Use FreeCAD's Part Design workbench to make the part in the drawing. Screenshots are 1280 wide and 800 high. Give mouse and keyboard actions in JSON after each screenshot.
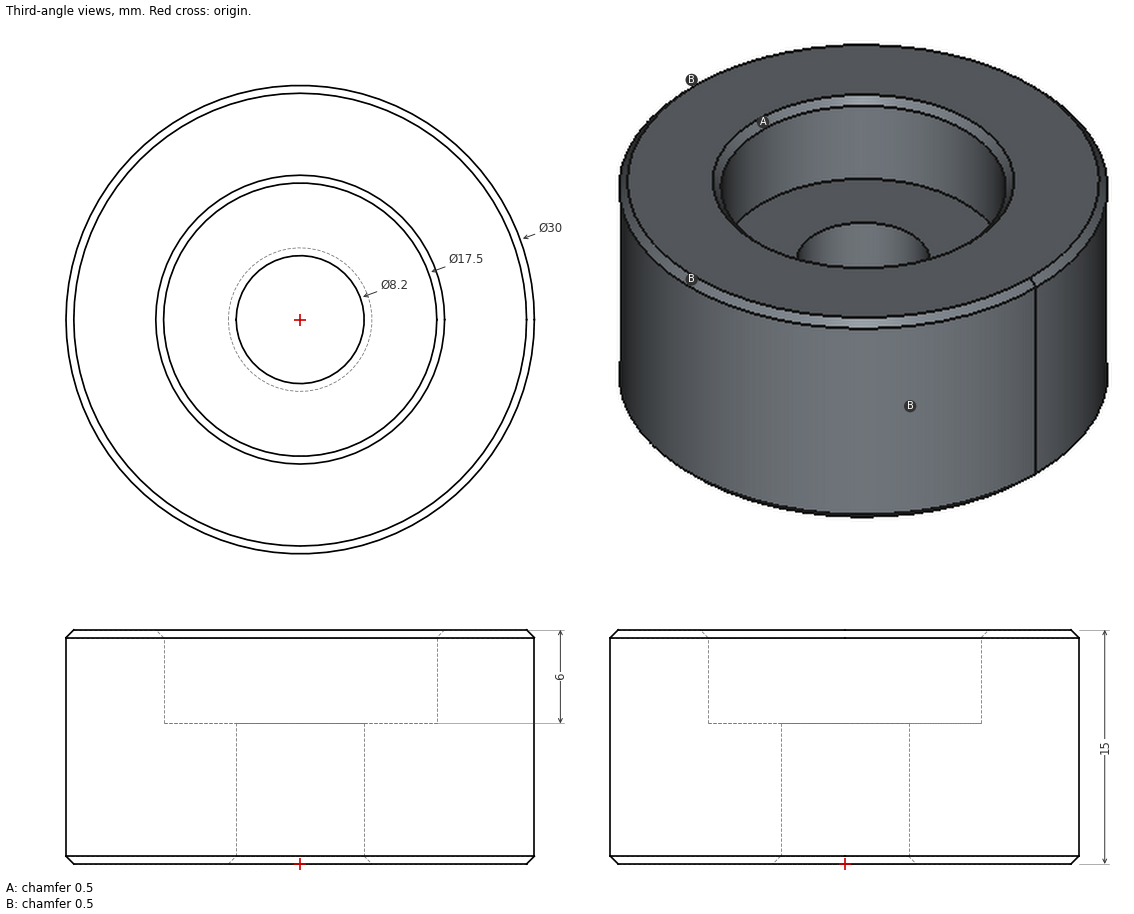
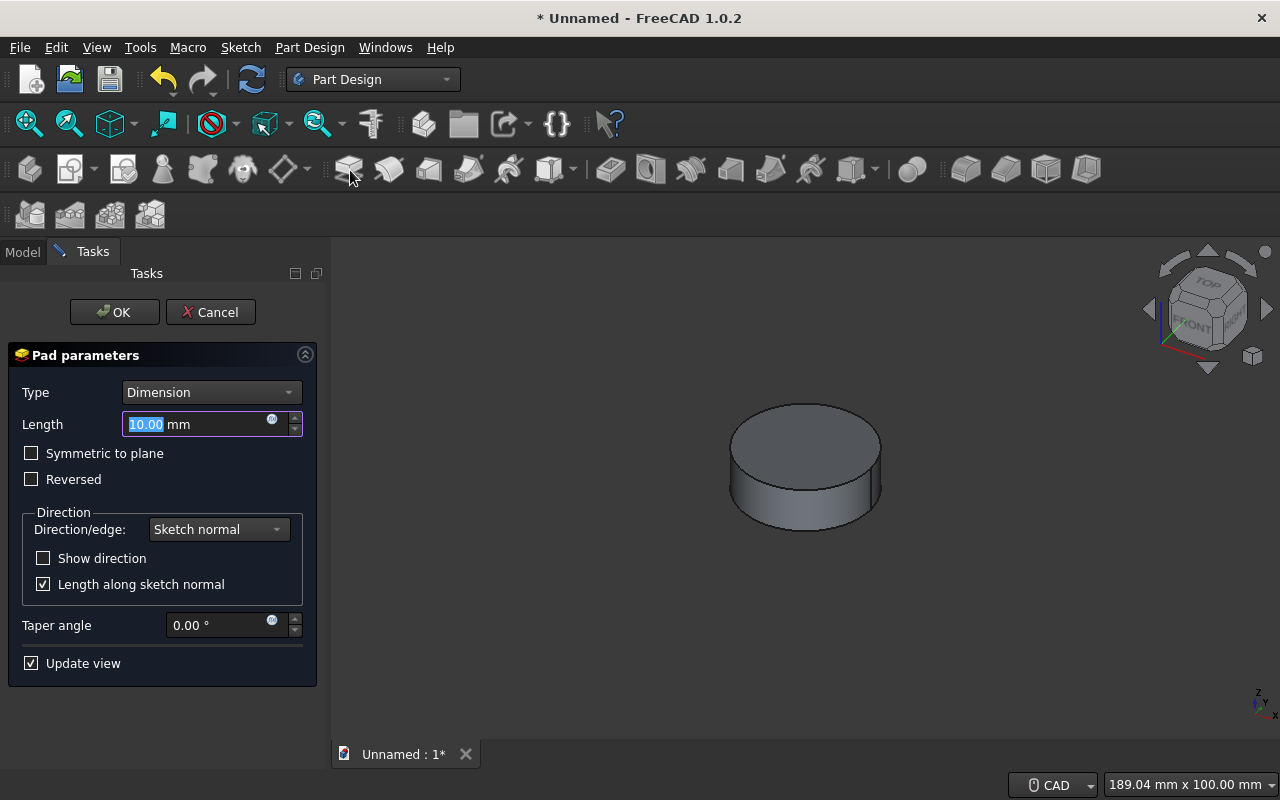
{"action": "type", "text": "15"}
{"action": "key", "text": "Tab"}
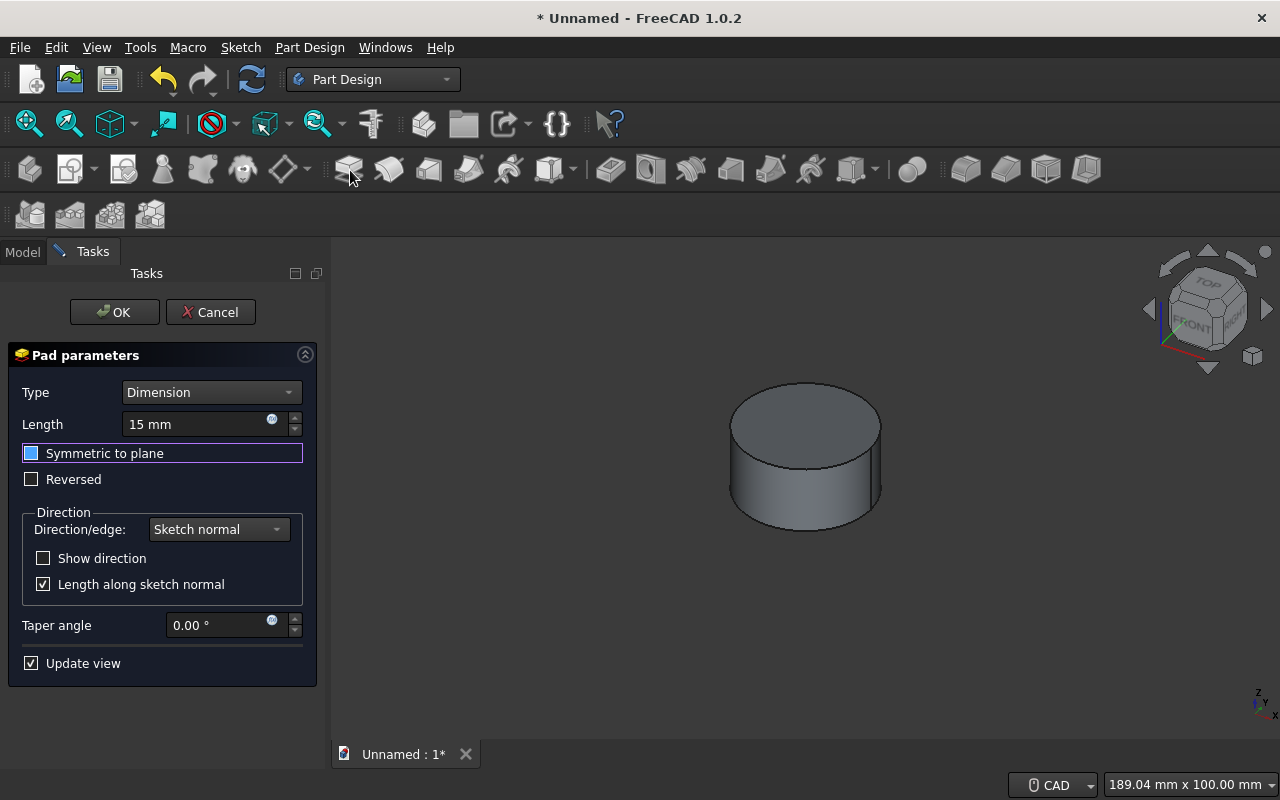
{"action": "left_click", "coordinate": [115, 312]}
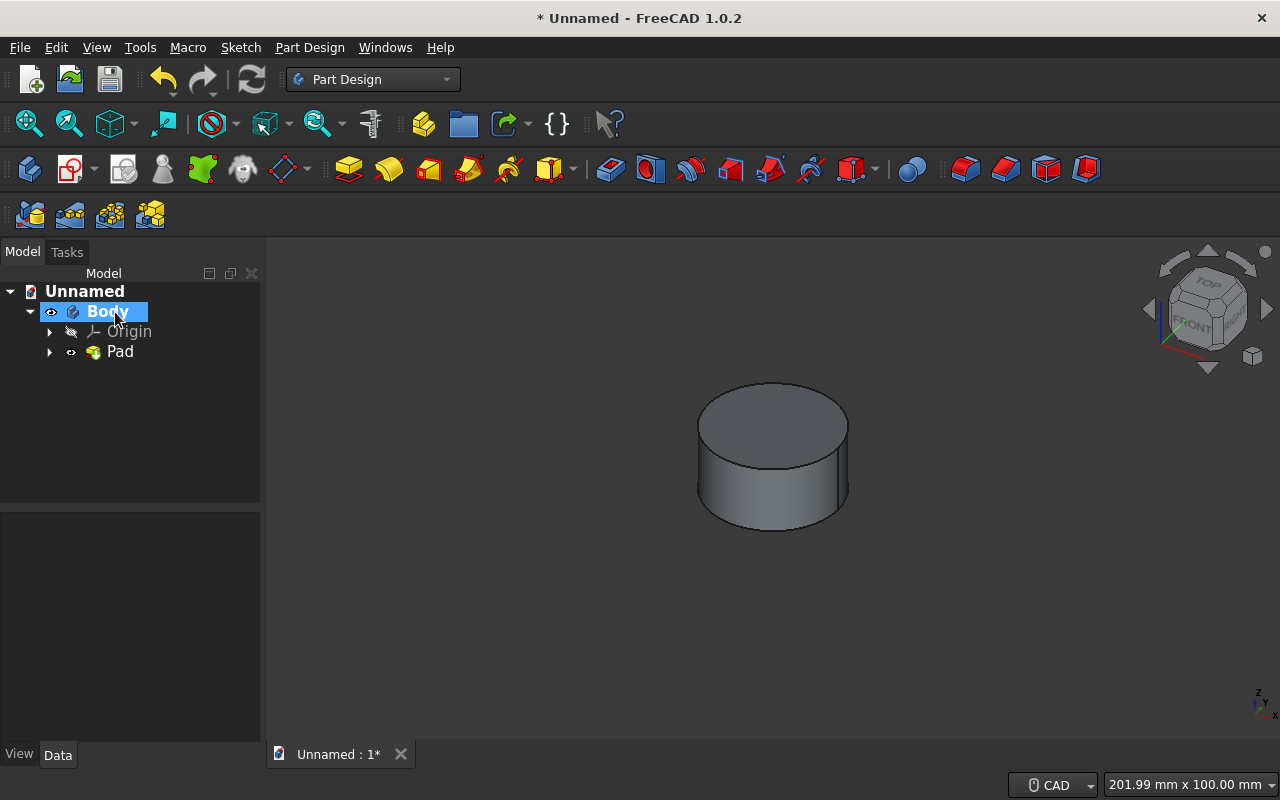
{"action": "left_click", "coordinate": [30, 124]}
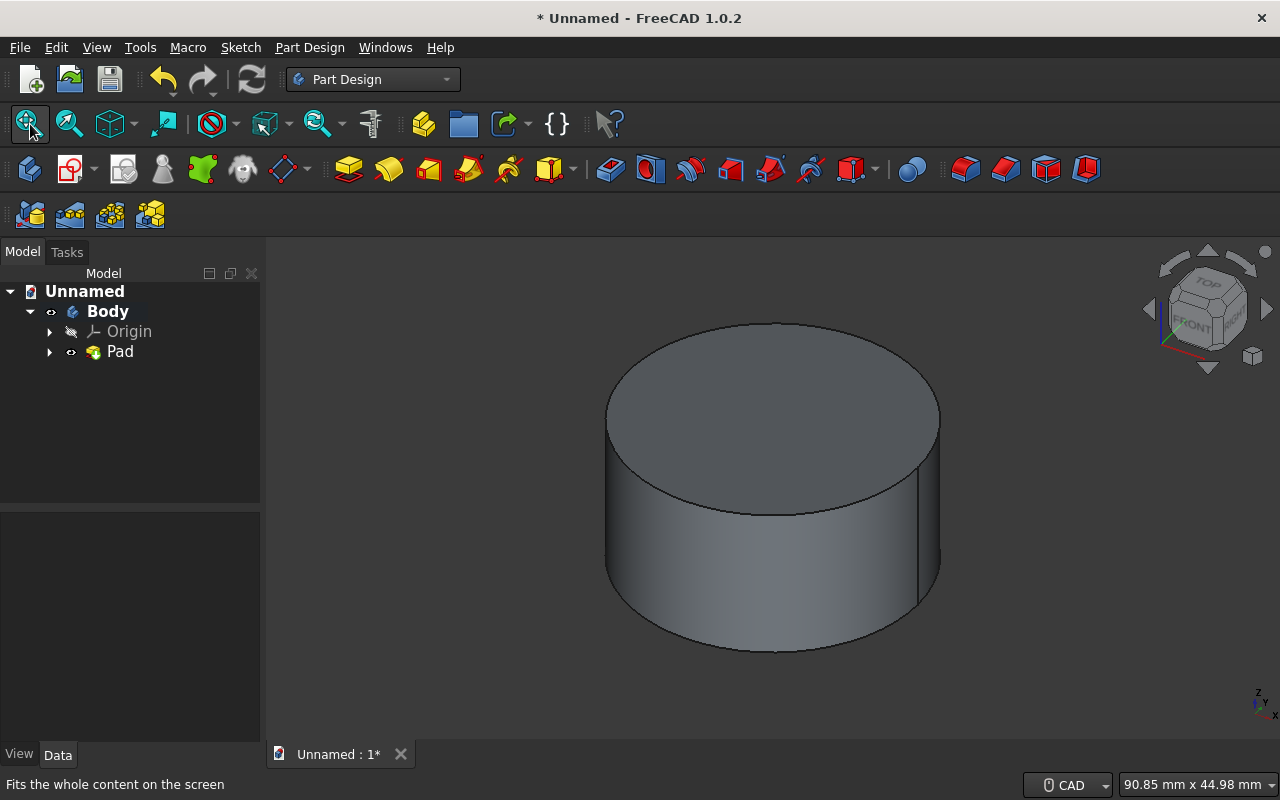
{"action": "left_click", "coordinate": [70, 170]}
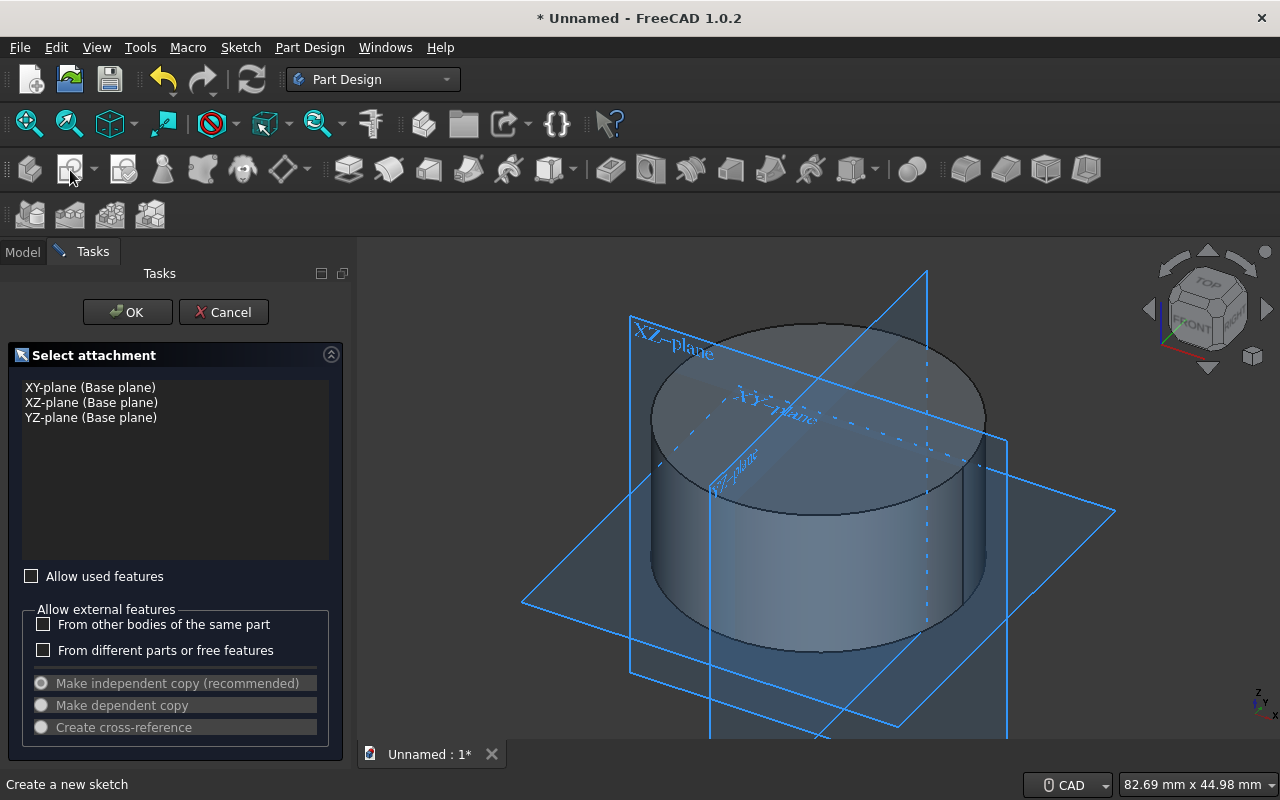
{"action": "left_click", "coordinate": [82, 388]}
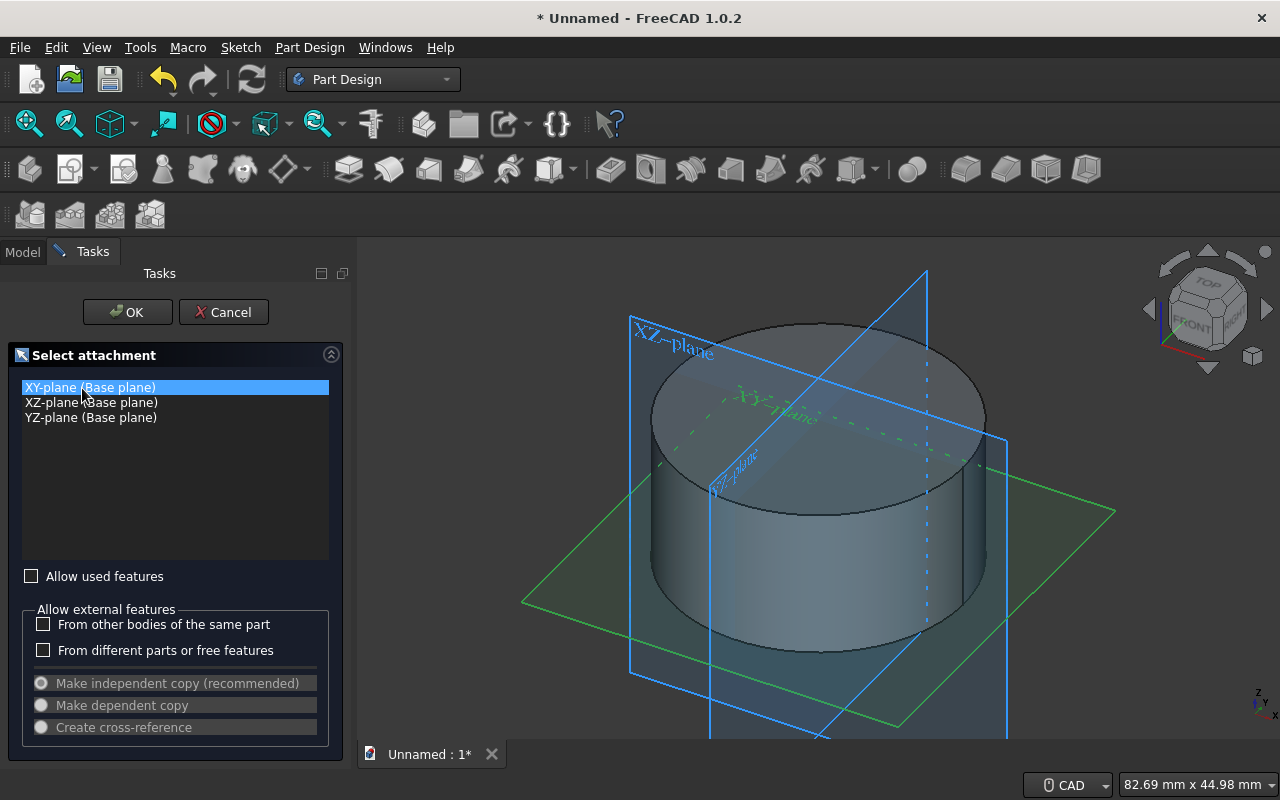
{"action": "left_click", "coordinate": [128, 312]}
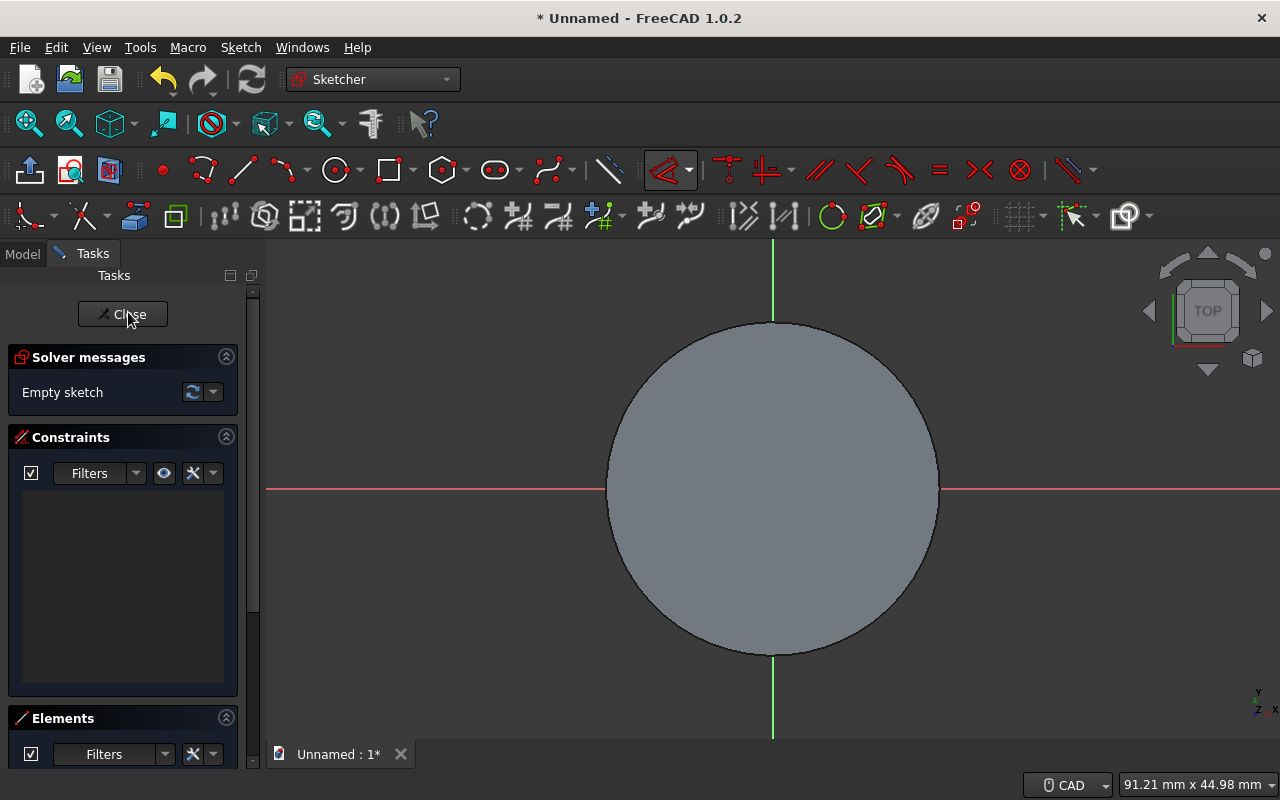
{"action": "key", "text": "q s"}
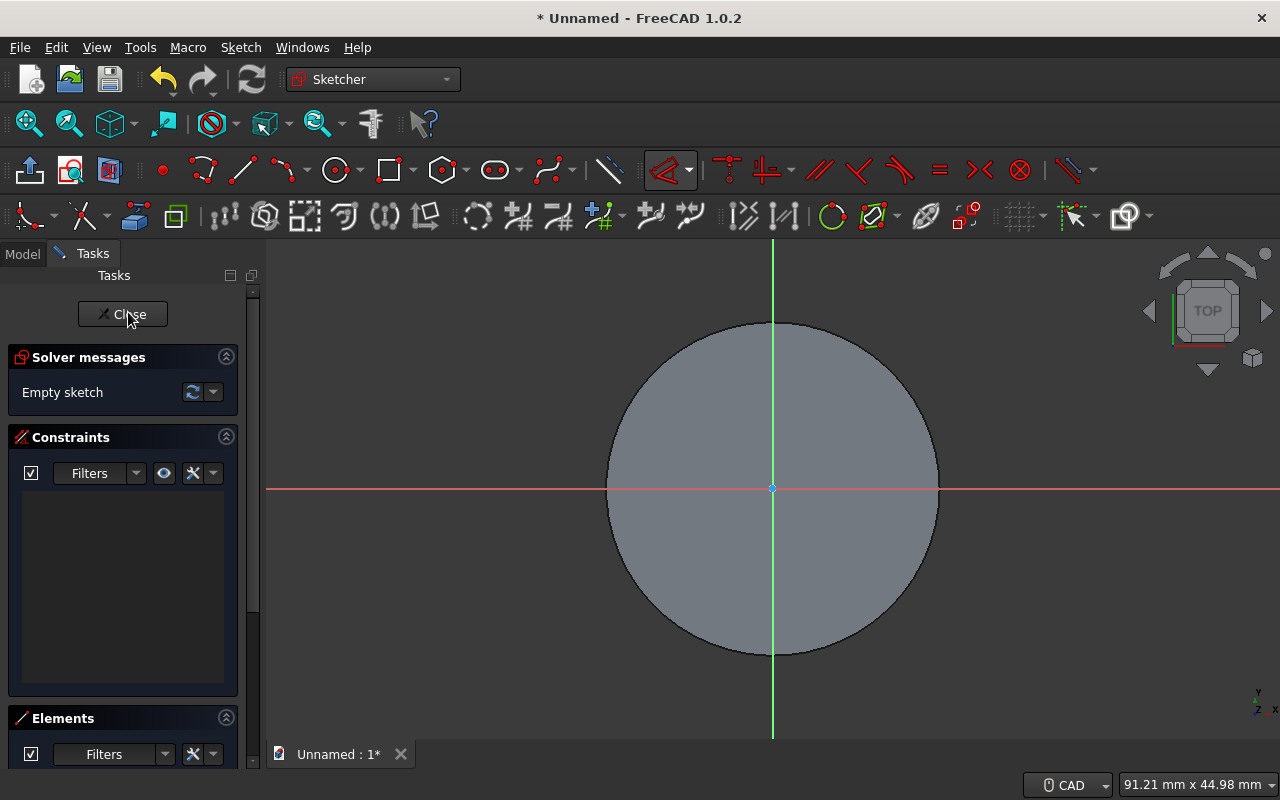
{"action": "scroll", "coordinate": [802, 489], "scroll_direction": "up", "scroll_amount": 6}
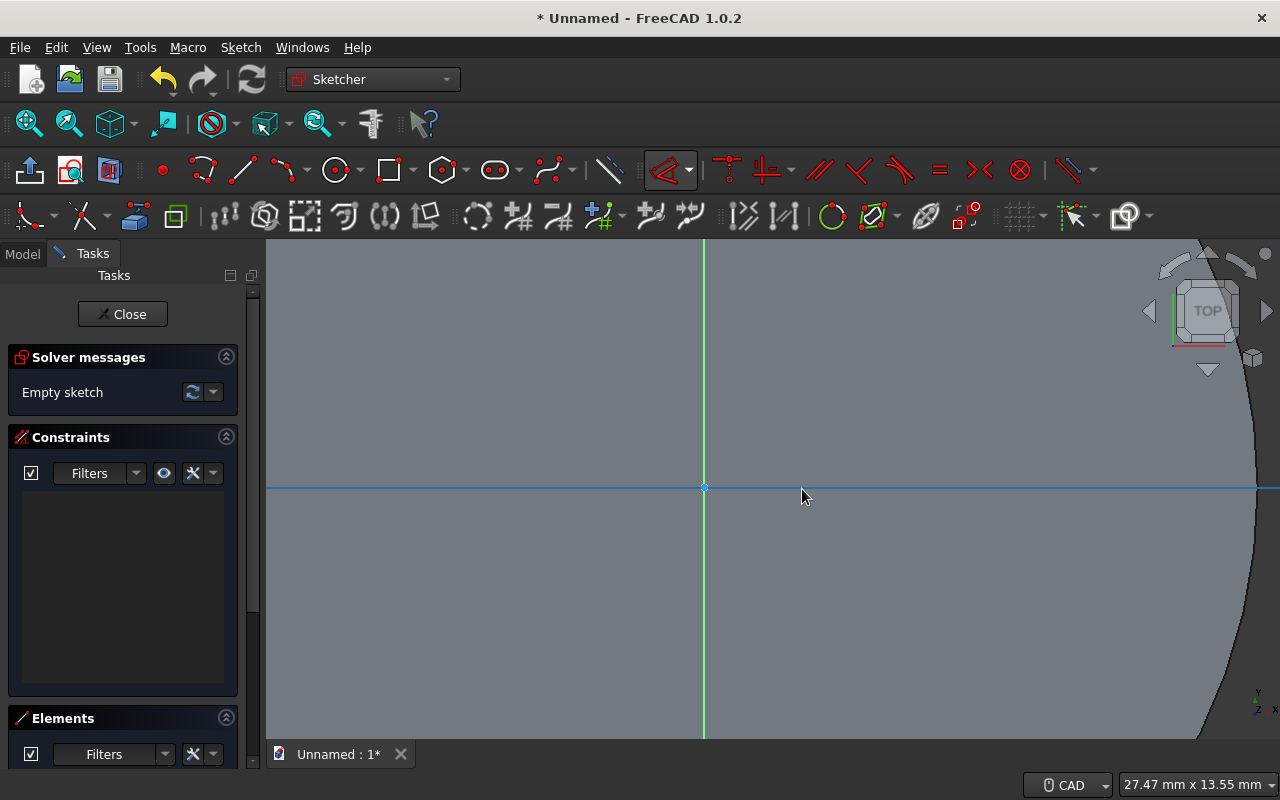
{"action": "left_click", "coordinate": [336, 170]}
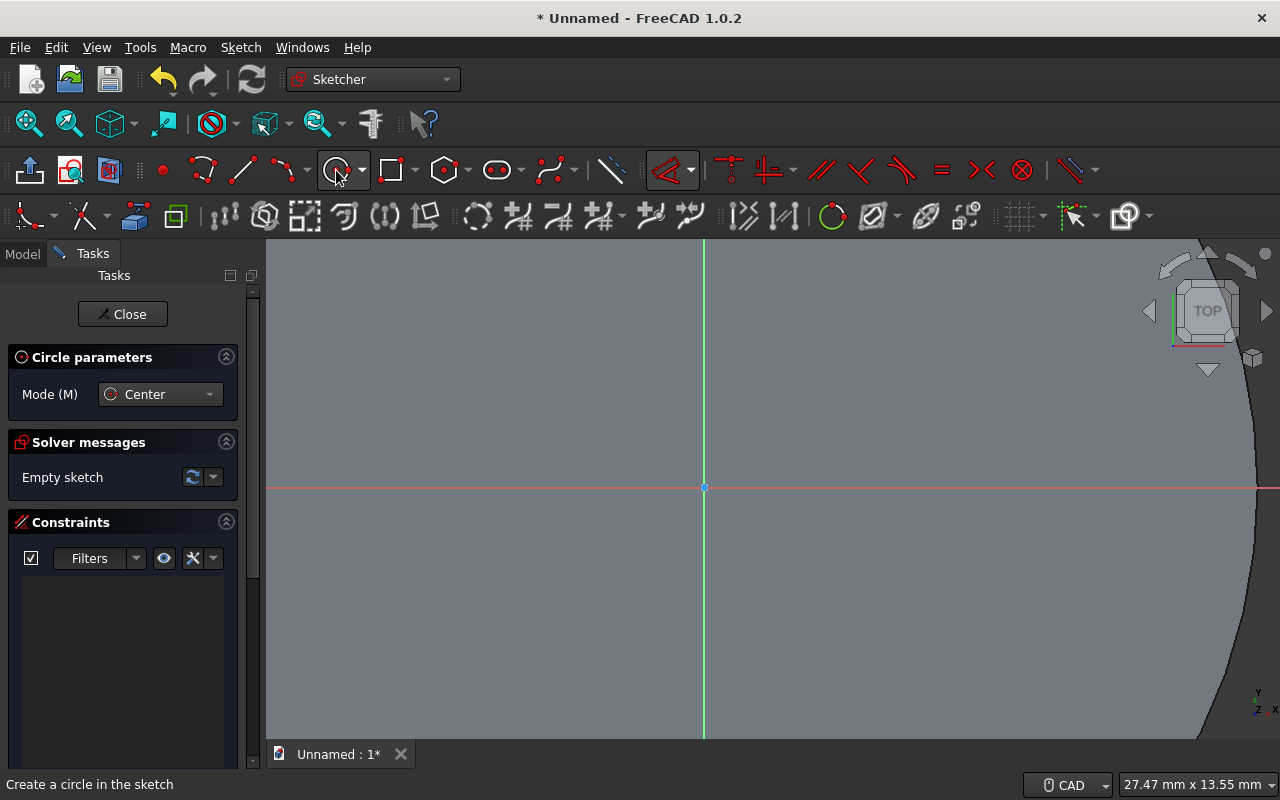
{"action": "left_click", "coordinate": [704, 488]}
{"action": "mouse_move", "coordinate": [811, 381]}